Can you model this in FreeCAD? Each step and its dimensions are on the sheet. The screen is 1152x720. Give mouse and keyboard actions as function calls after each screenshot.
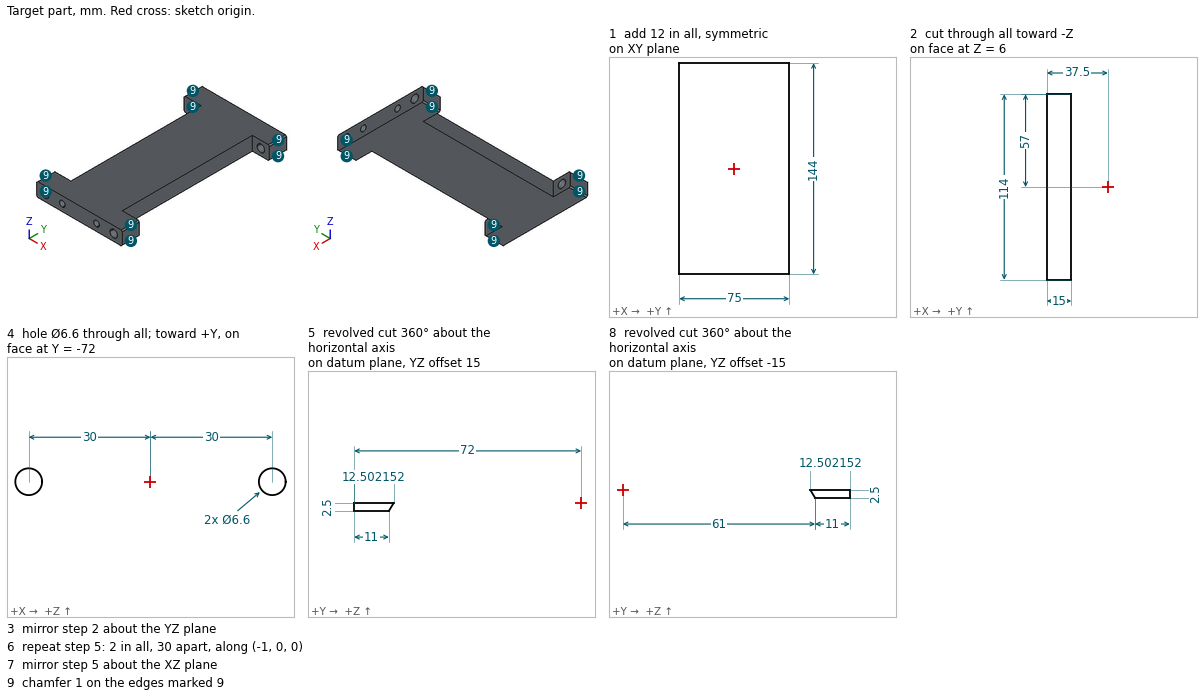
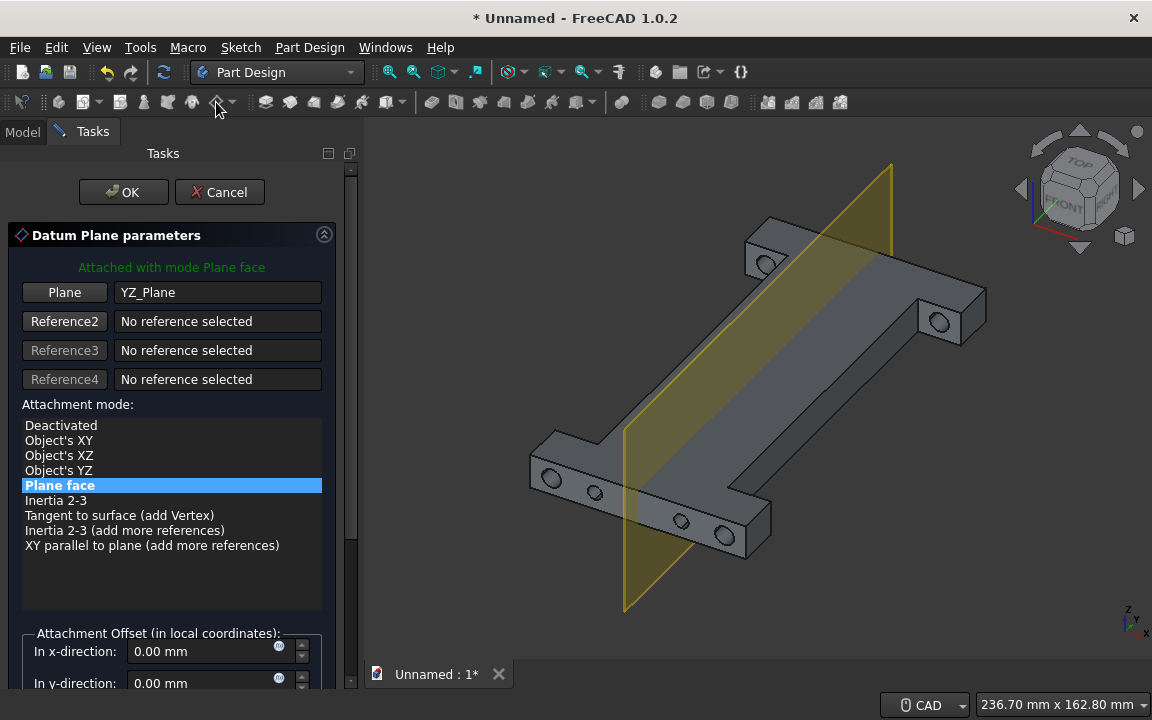
scroll(351, 426, down, 2)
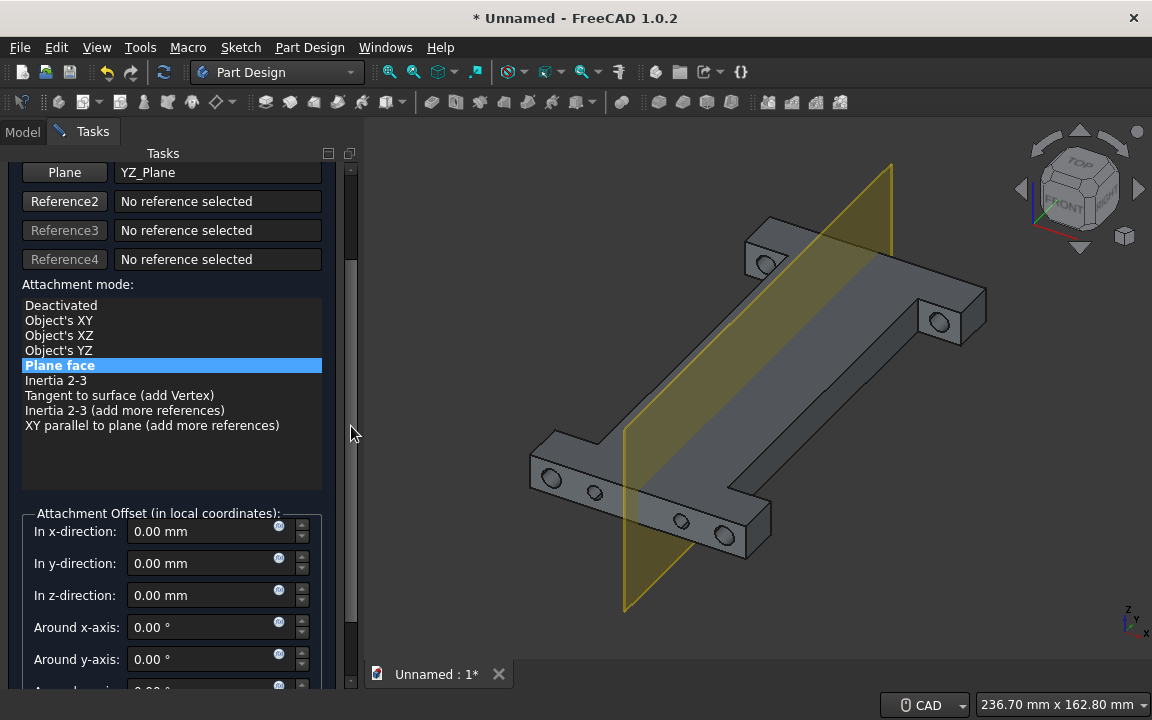
triple_click(210, 595)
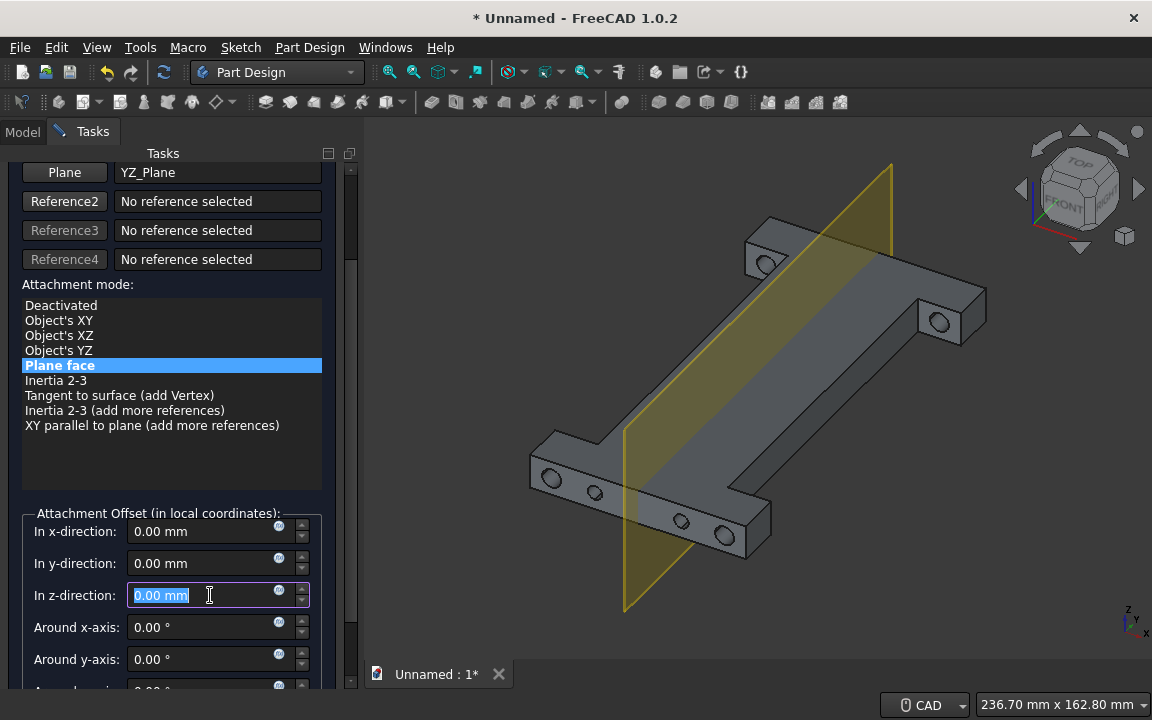
text(-15)
key(Tab)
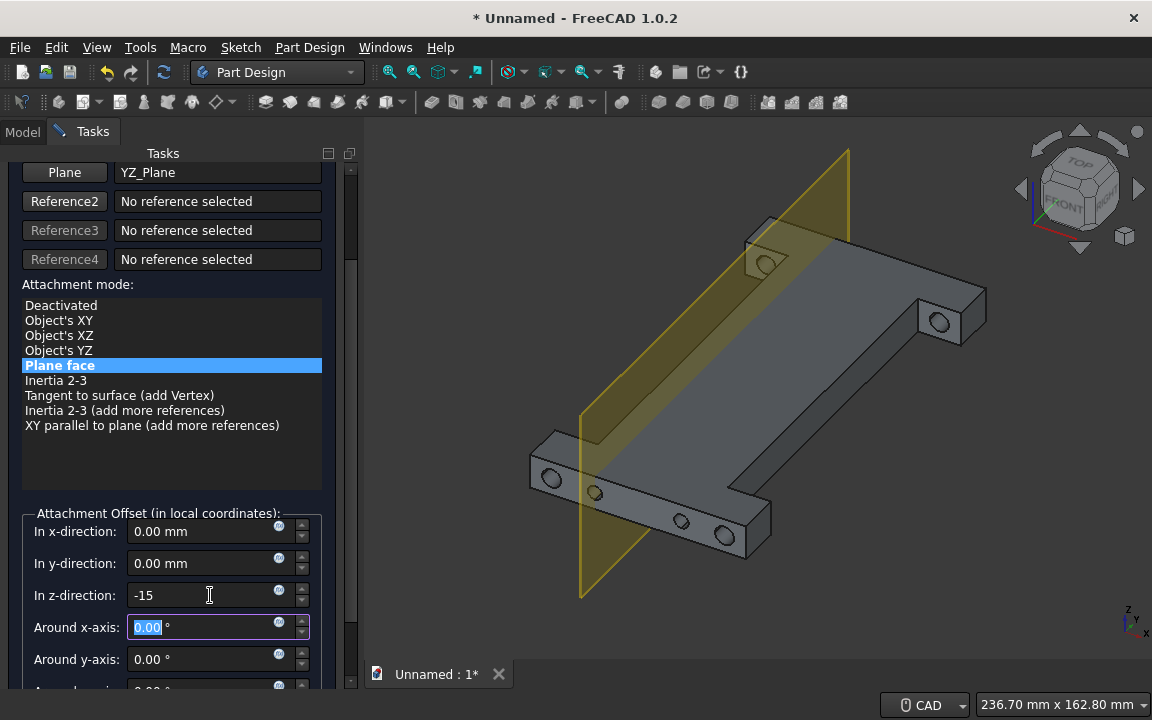
scroll(351, 426, up, 3)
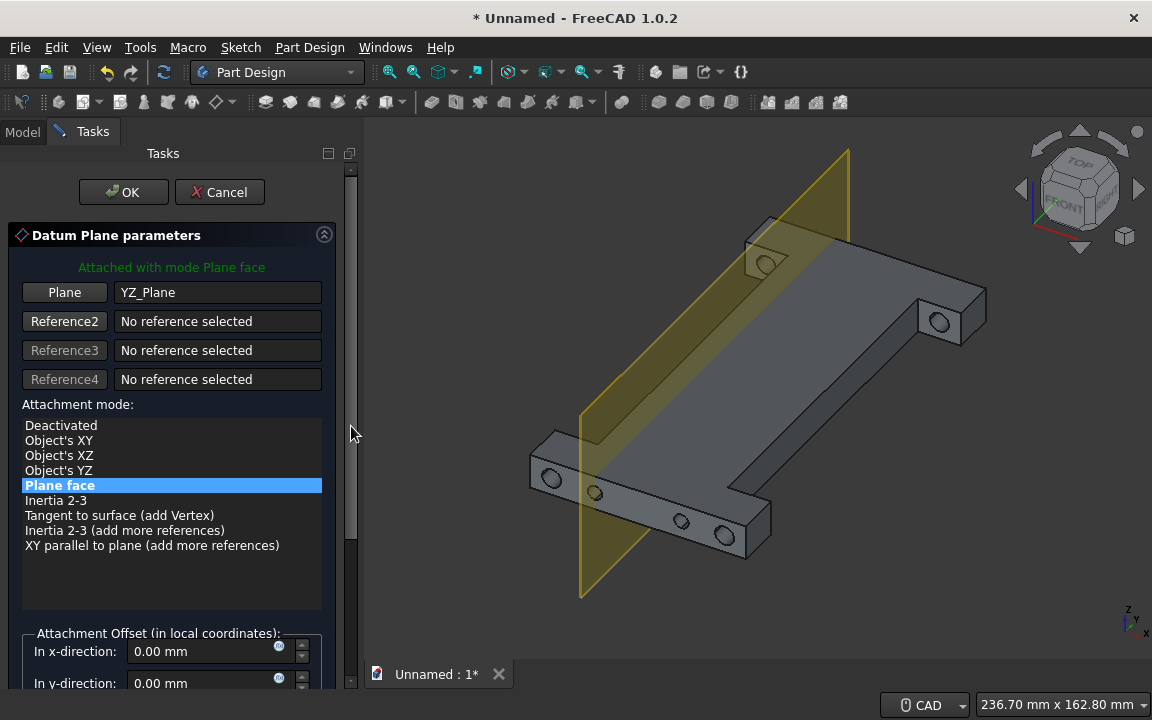
click(124, 192)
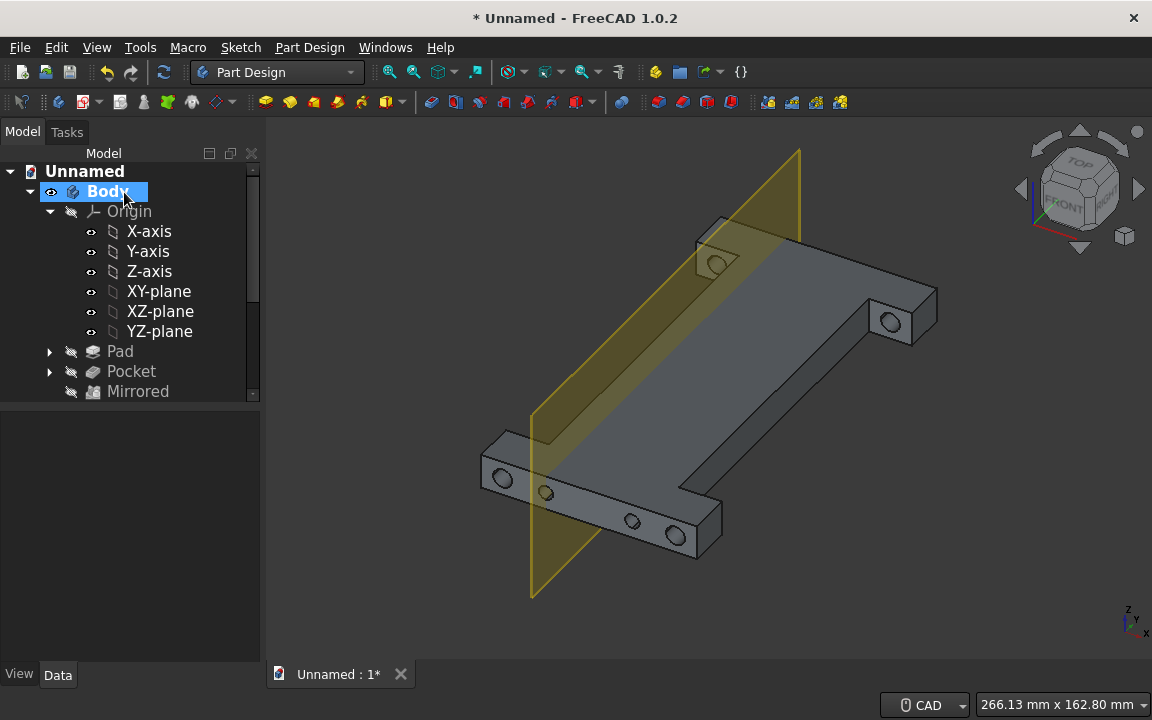
scroll(100, 287, down, 3)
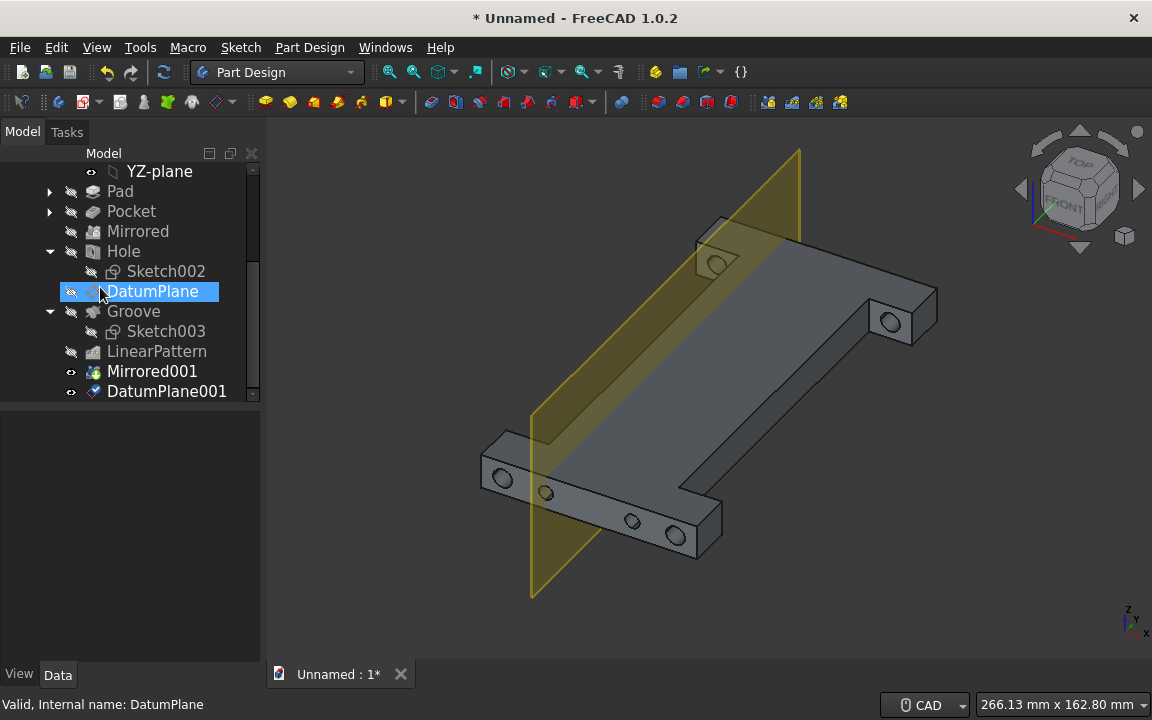
click(116, 392)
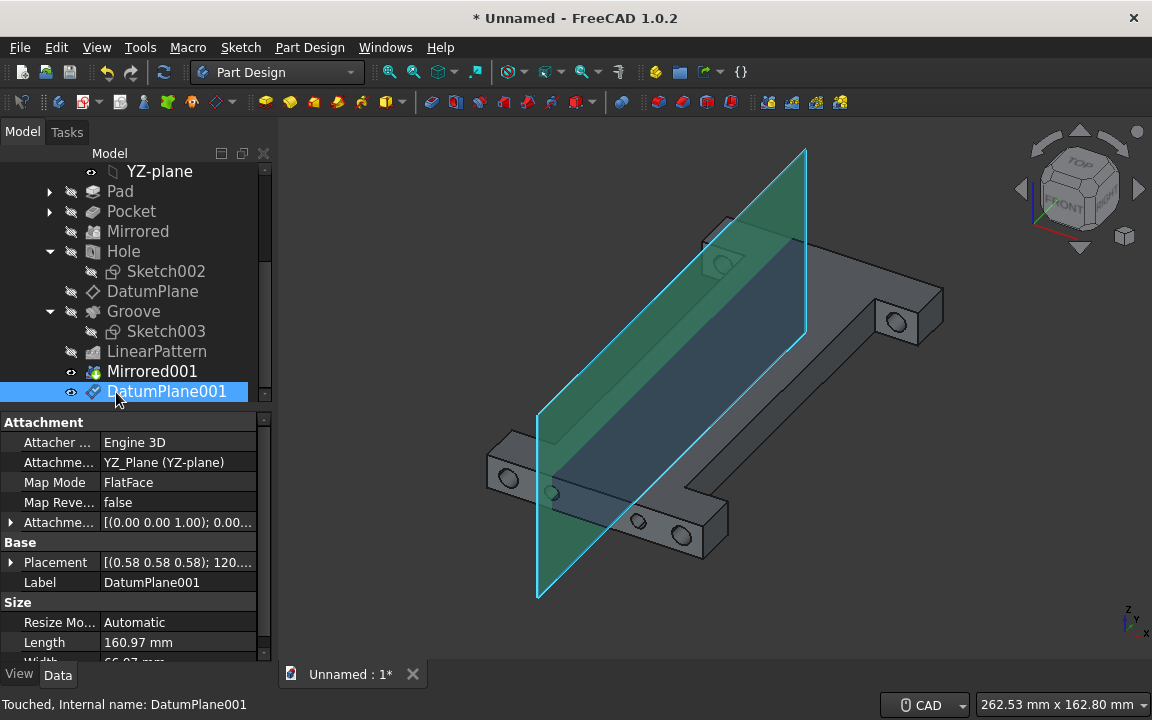
click(84, 102)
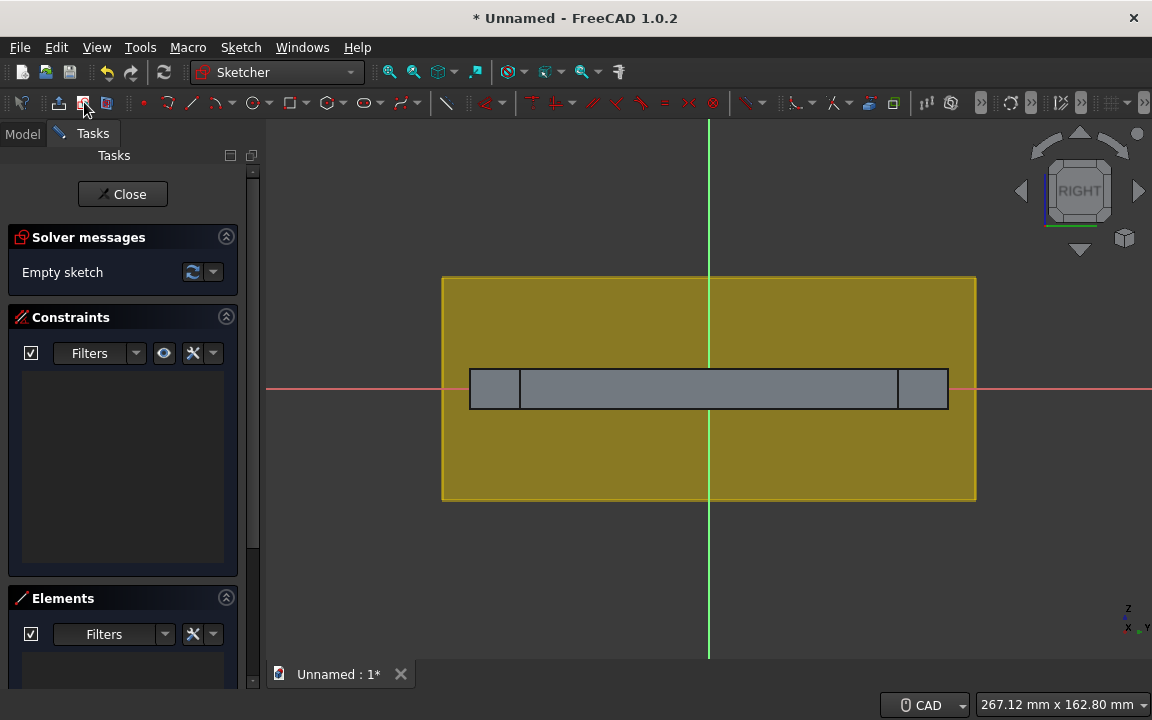
click(108, 104)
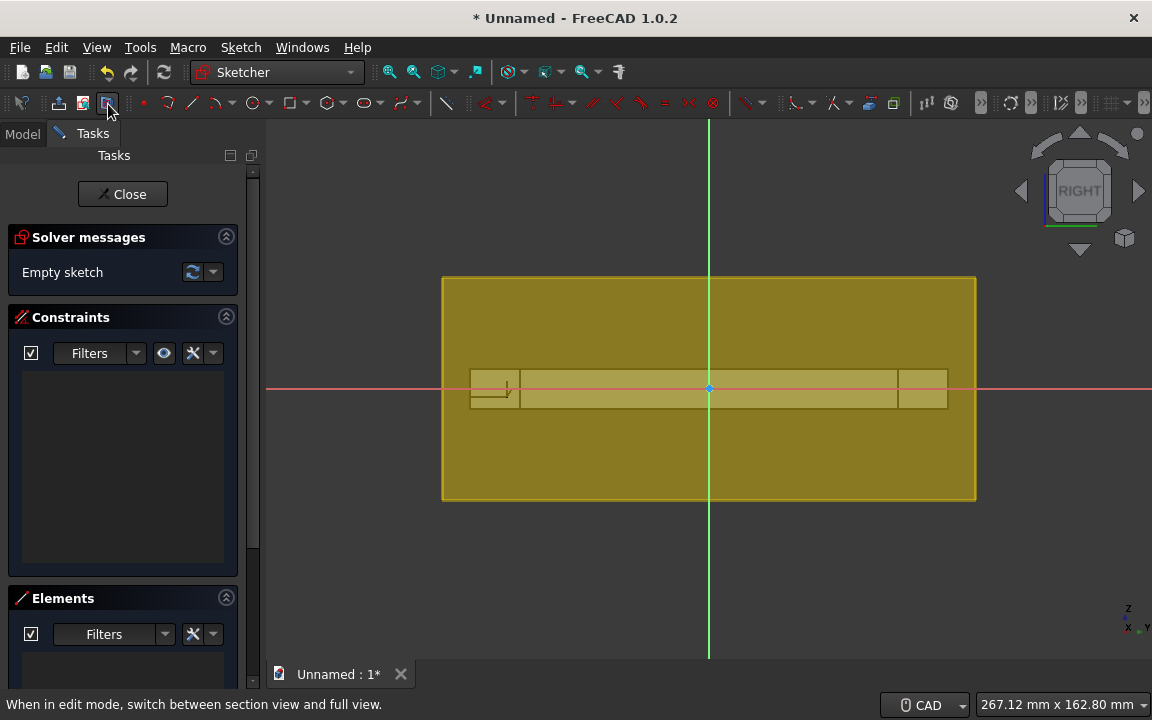
scroll(956, 394, up, 12)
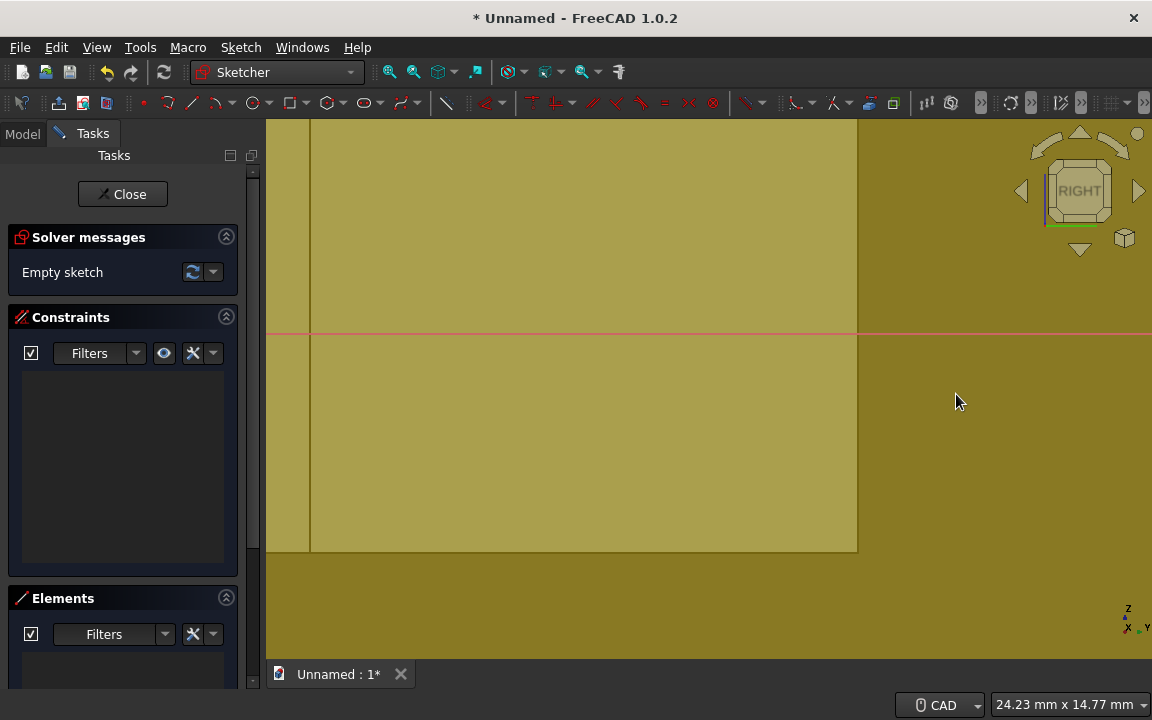
click(168, 104)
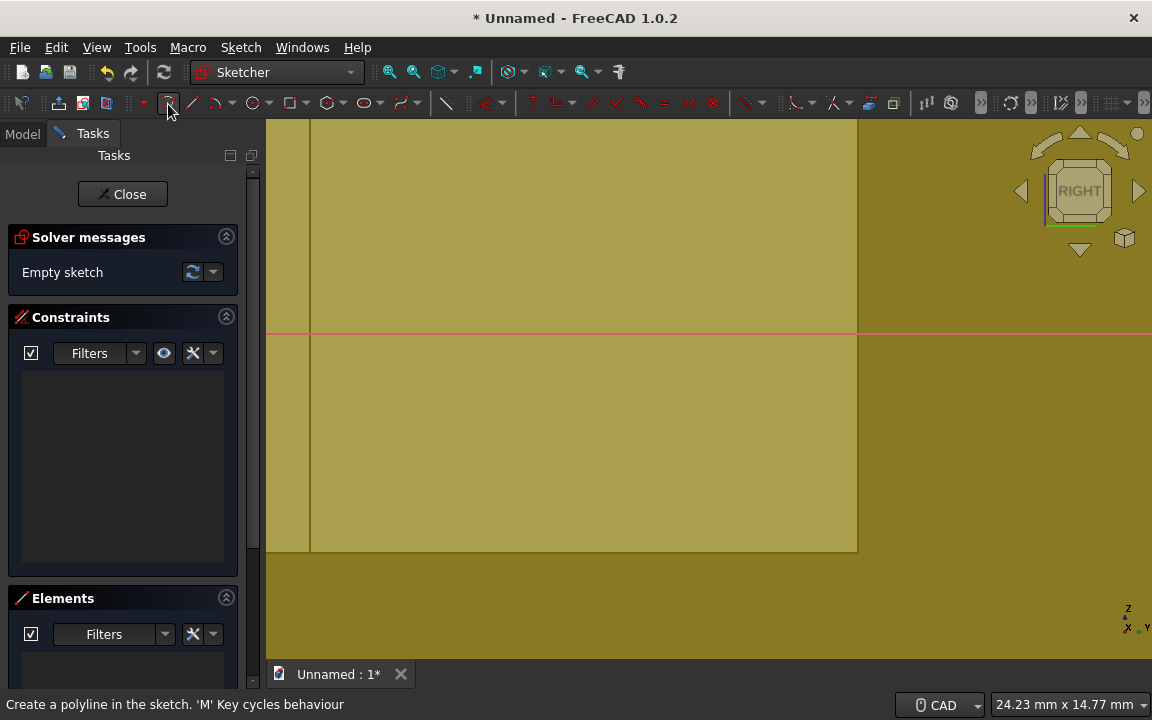
click(401, 334)
click(456, 425)
click(858, 425)
click(858, 343)
click(401, 334)
key(Escape)
key(Escape)